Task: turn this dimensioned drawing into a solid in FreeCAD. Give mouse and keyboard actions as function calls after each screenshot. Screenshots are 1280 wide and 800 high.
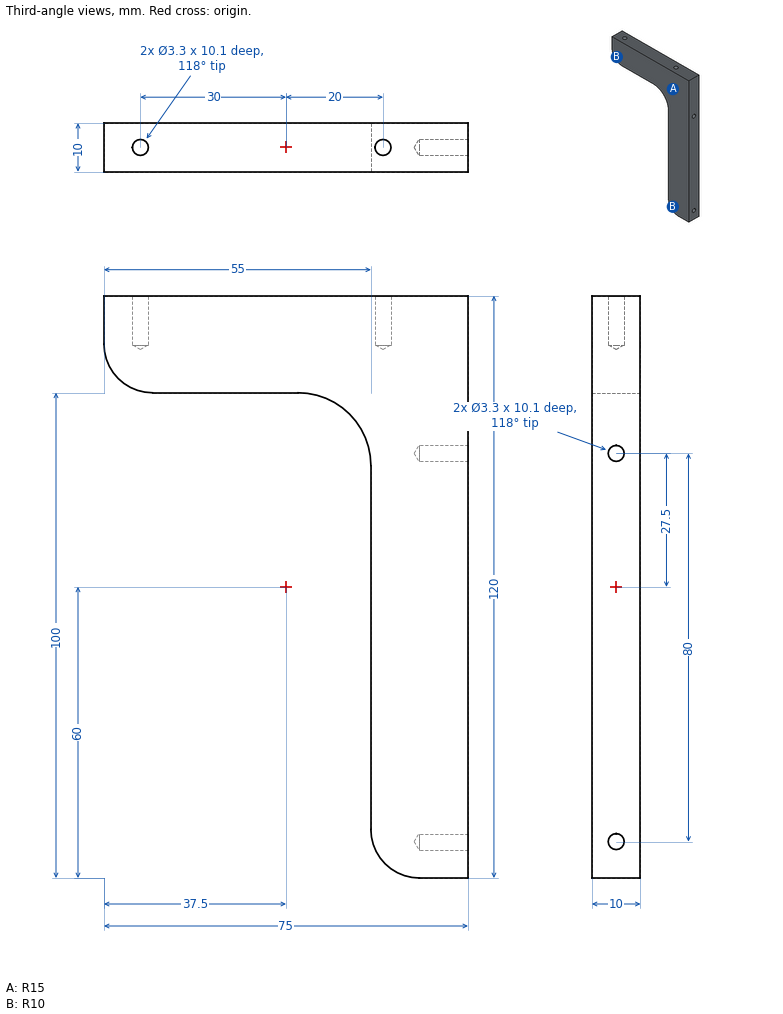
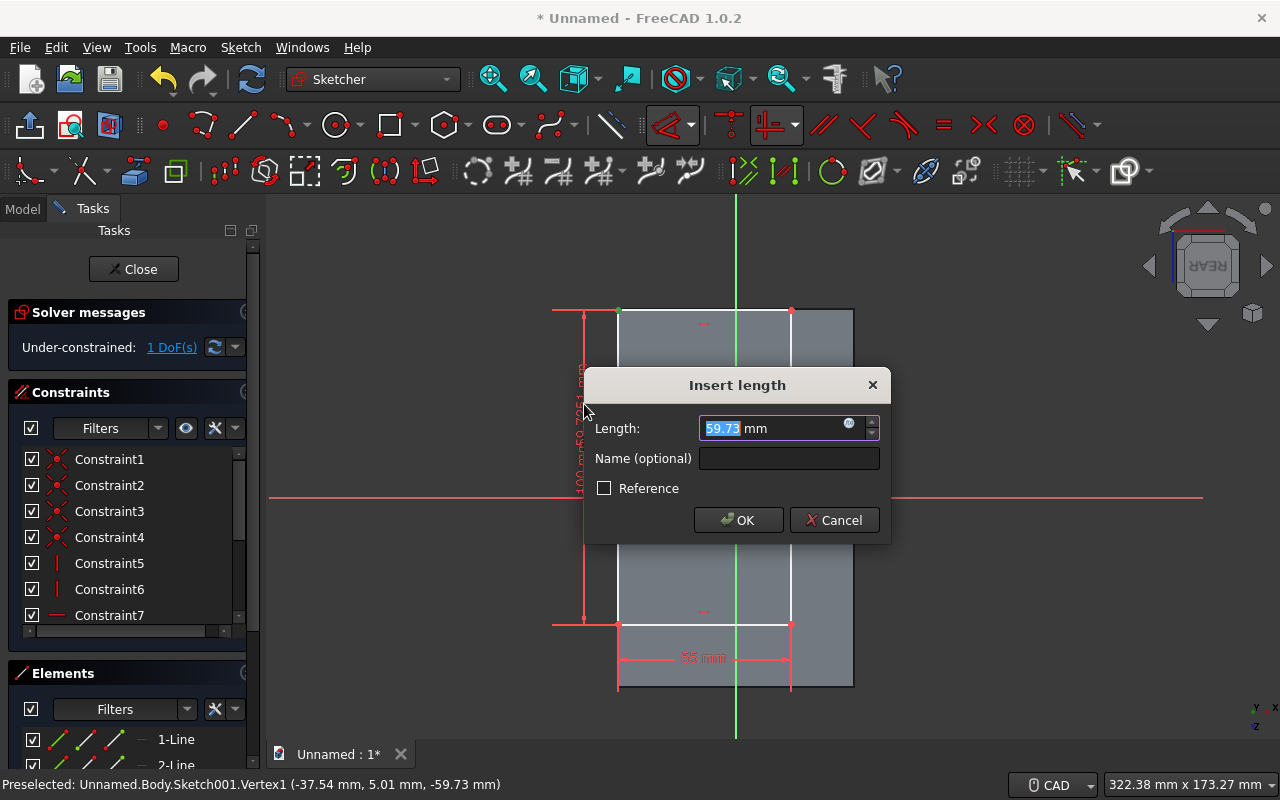
text(60)
key(Return)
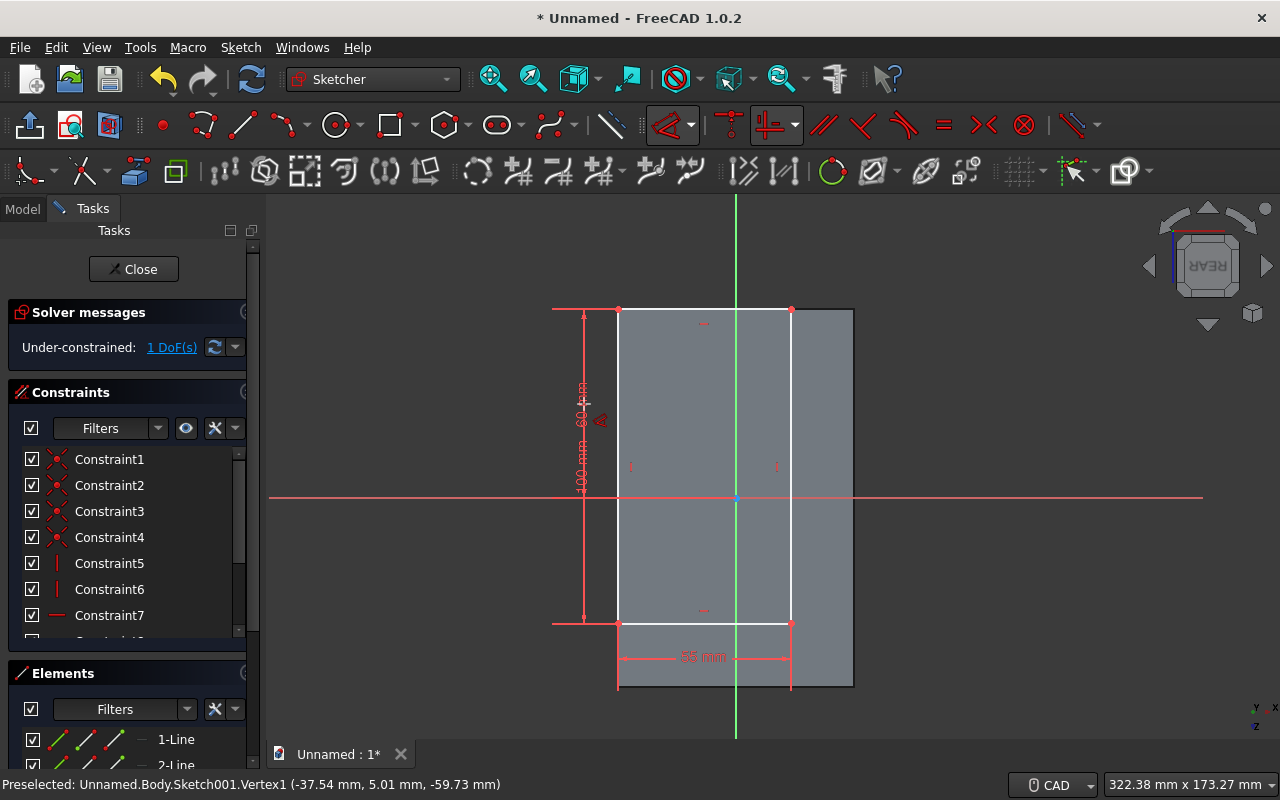
click(618, 309)
click(677, 275)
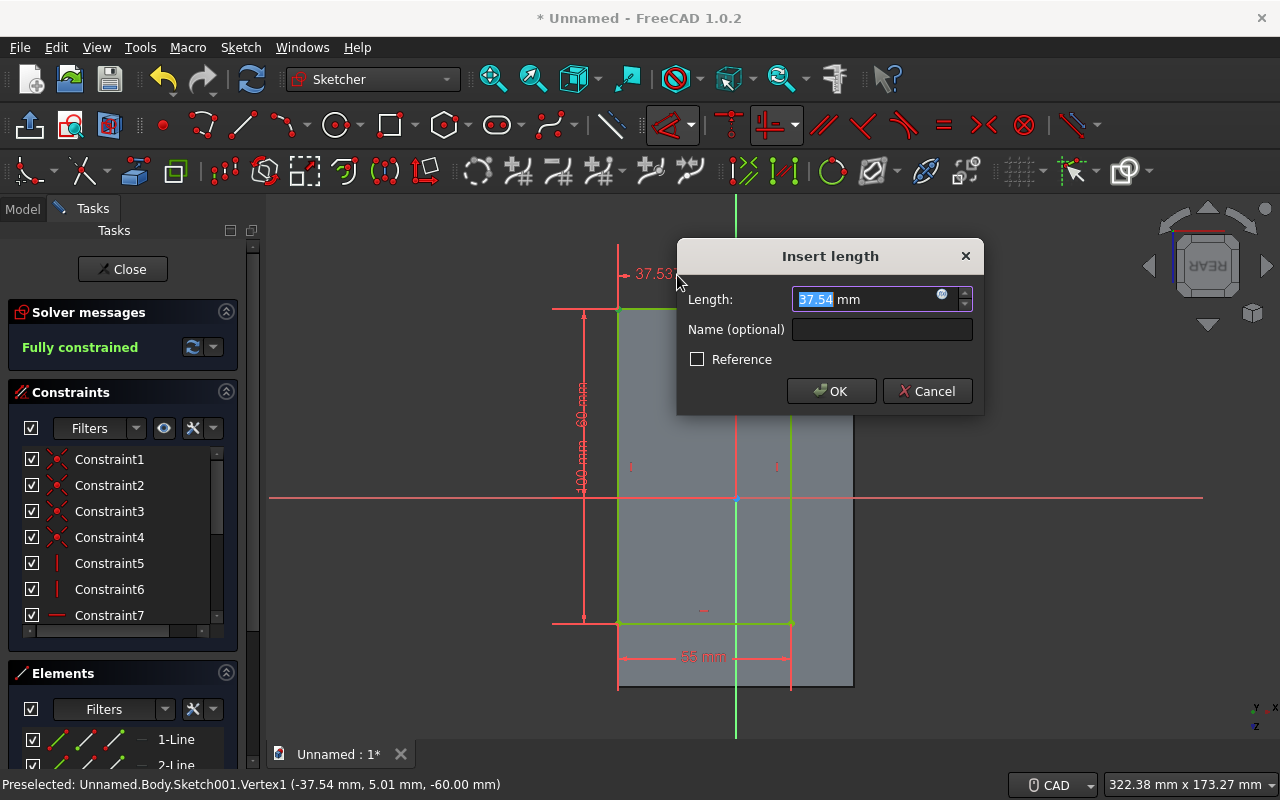
text(37.5)
key(Return)
key(Escape)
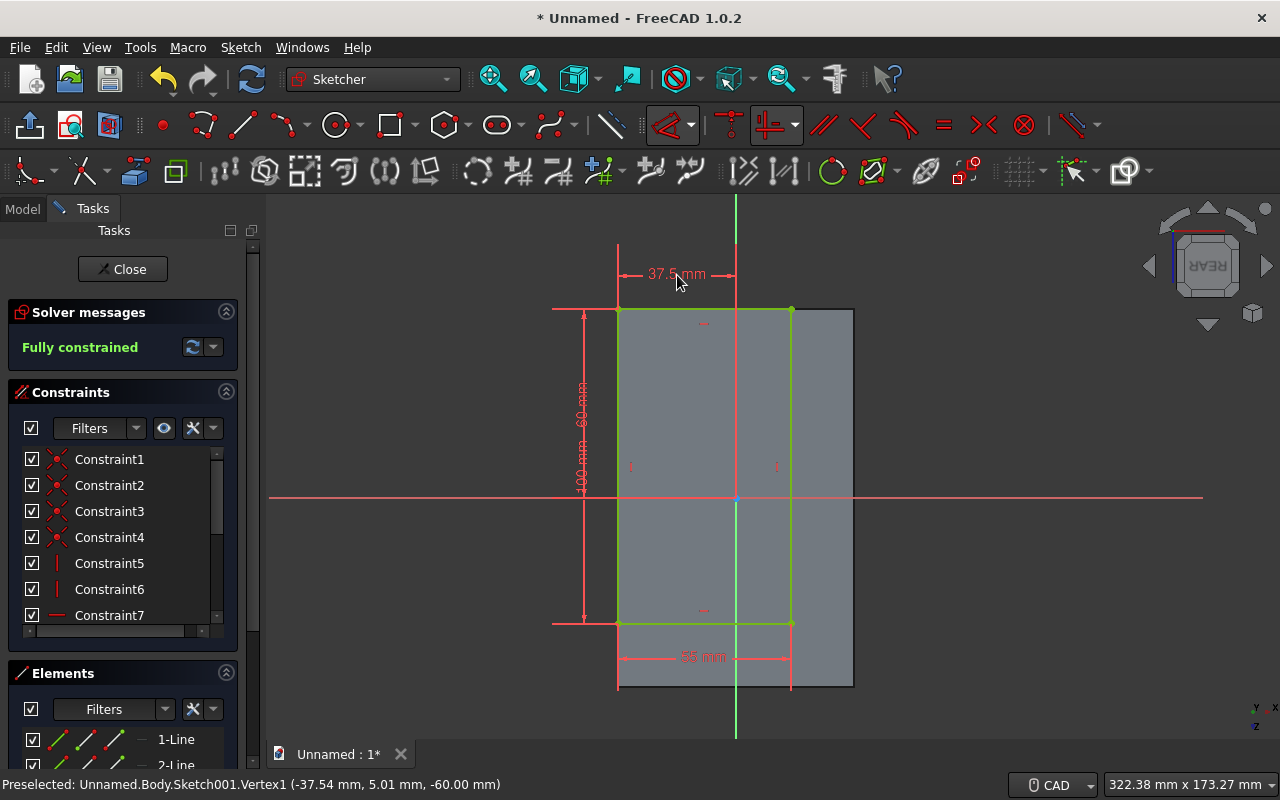
click(123, 269)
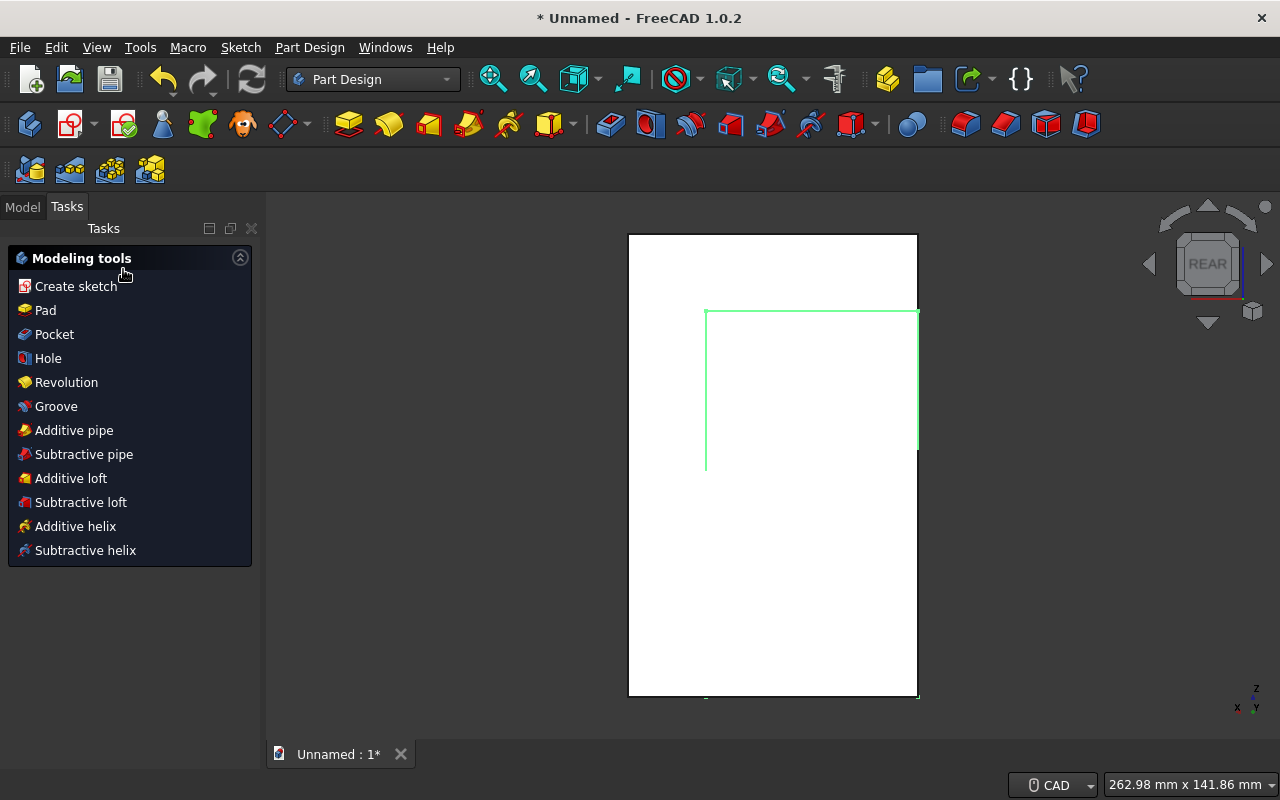
click(612, 124)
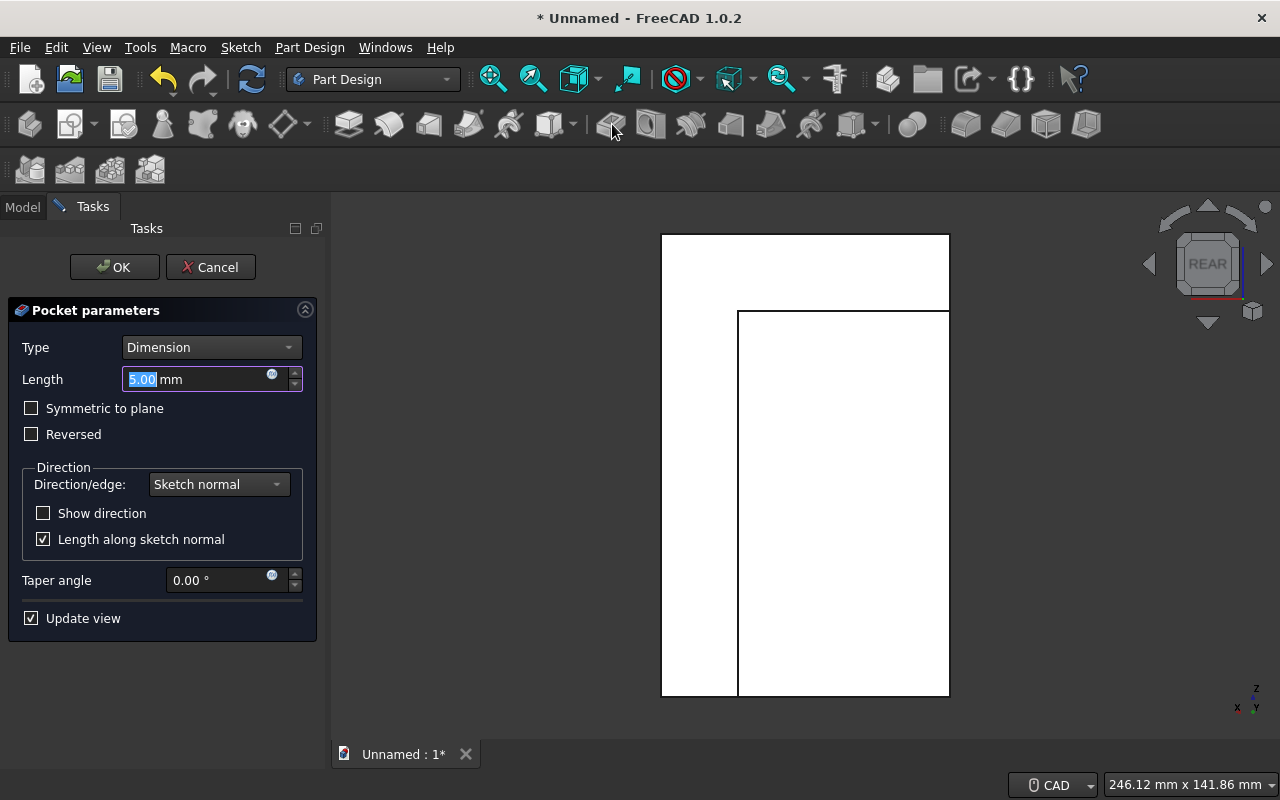
text(10)
key(Tab)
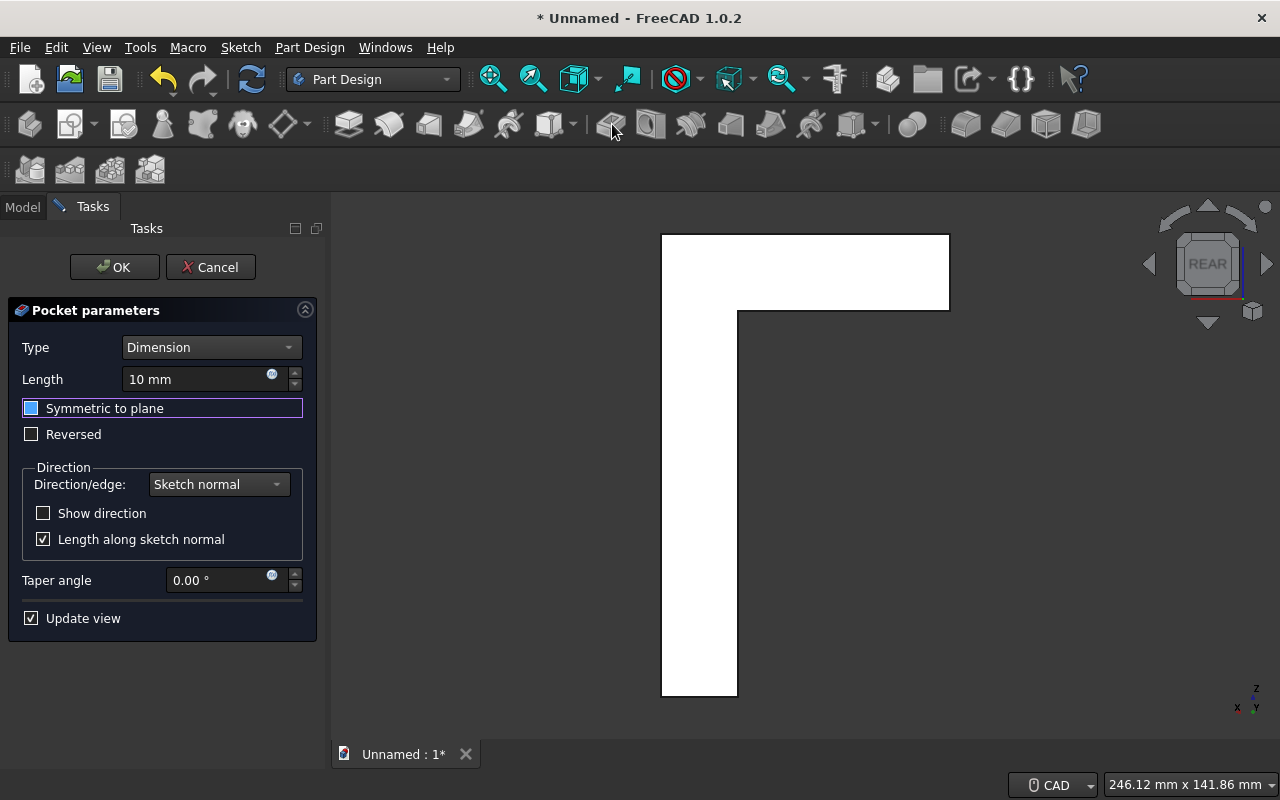
click(115, 267)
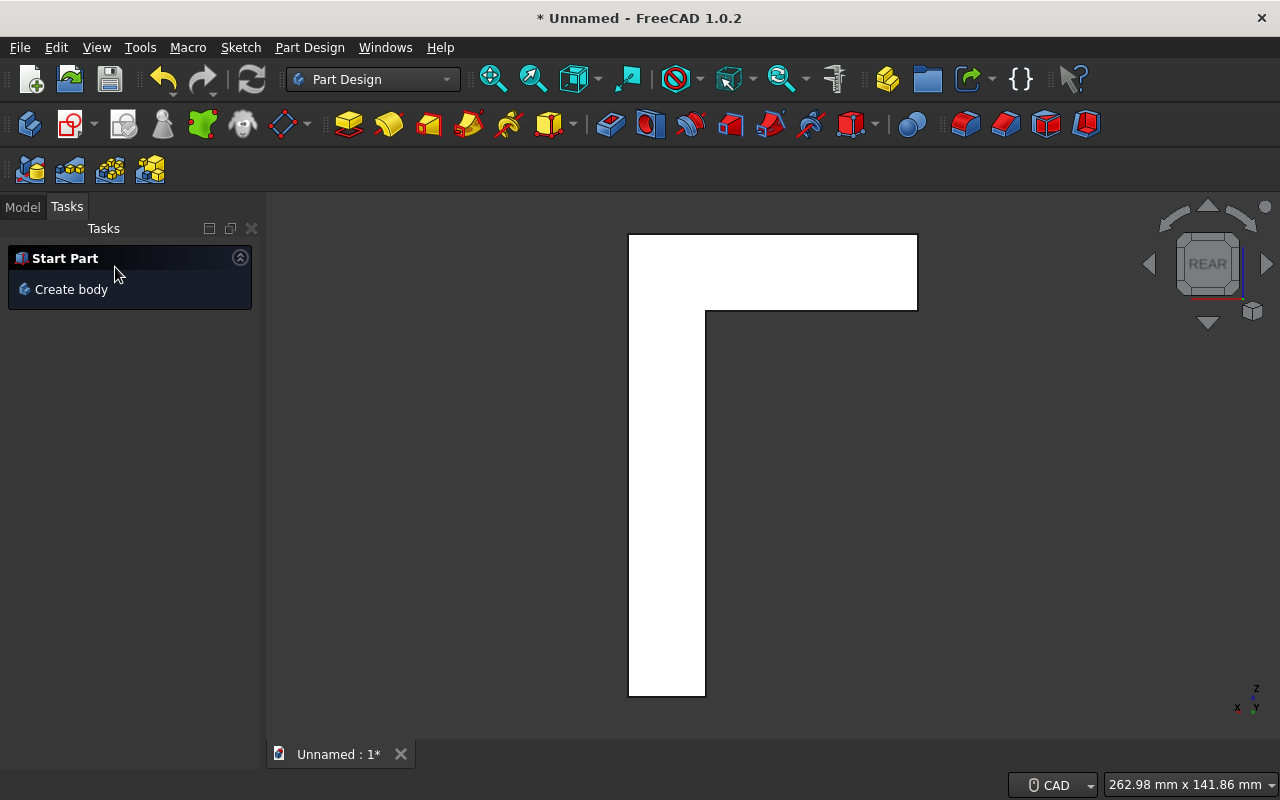
key(0)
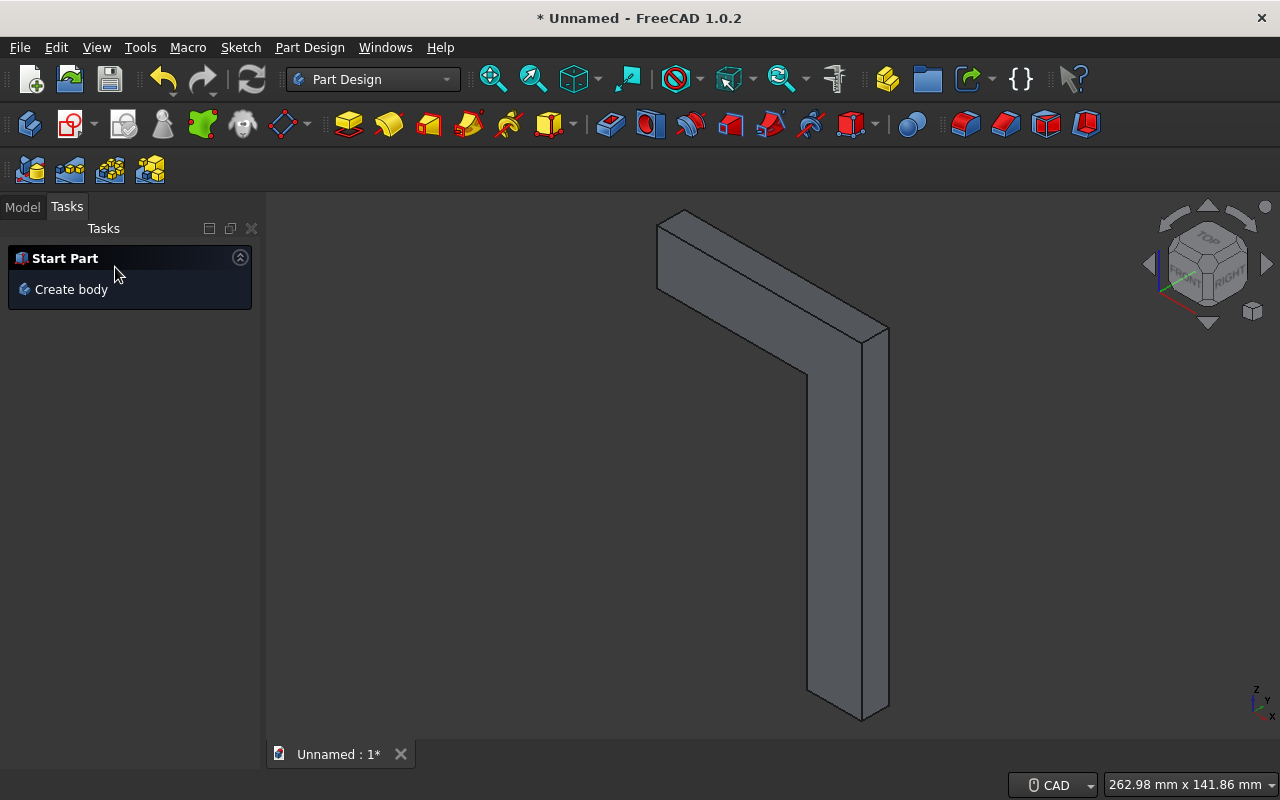
key(2)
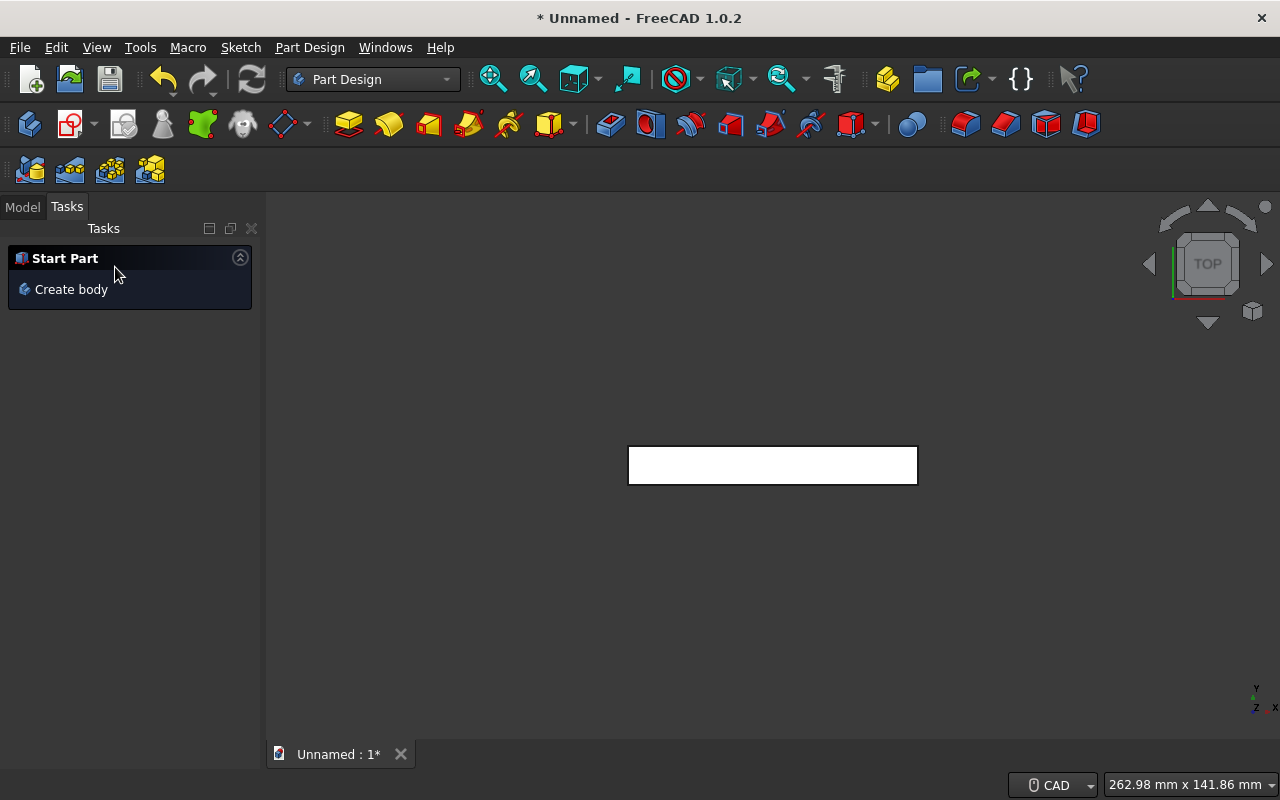
key(v)
key(f)